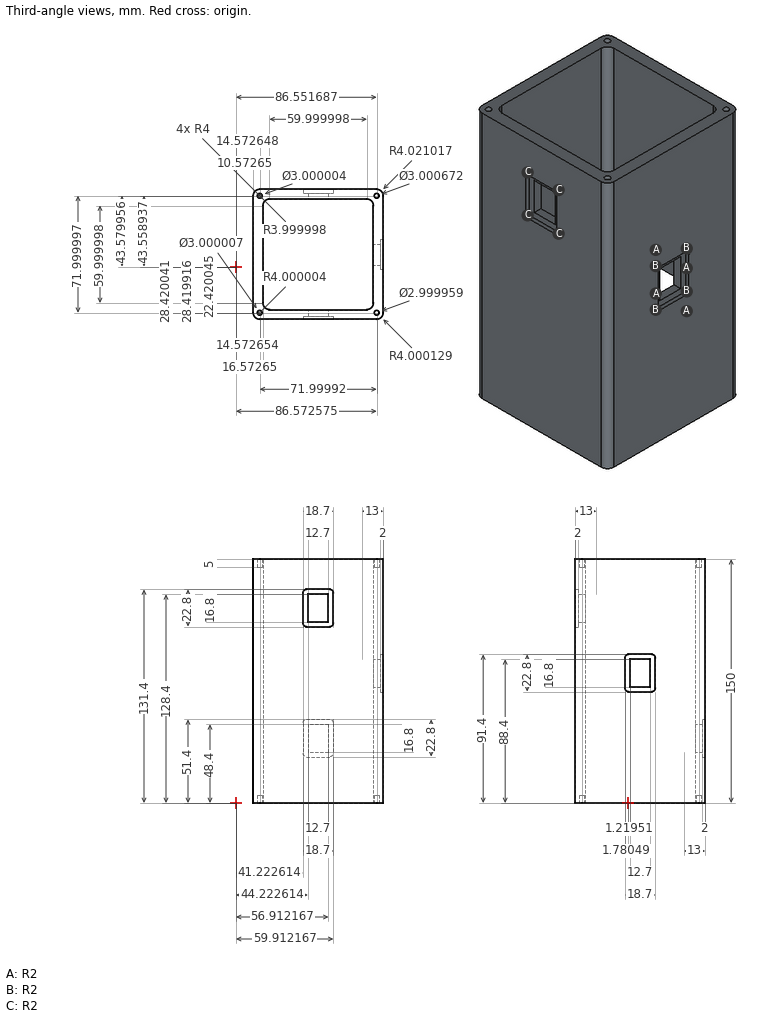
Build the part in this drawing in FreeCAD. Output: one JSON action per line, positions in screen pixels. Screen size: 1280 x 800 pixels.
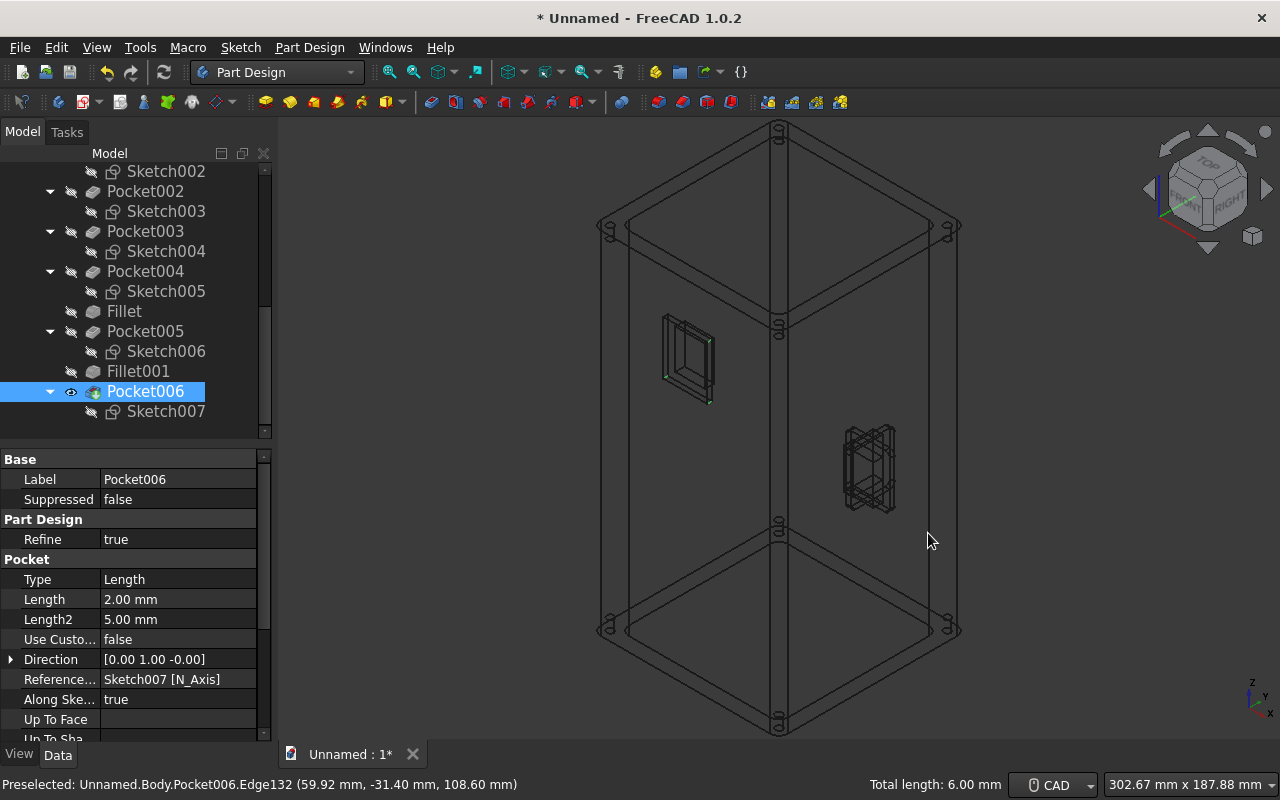
{"action": "key", "text": "2"}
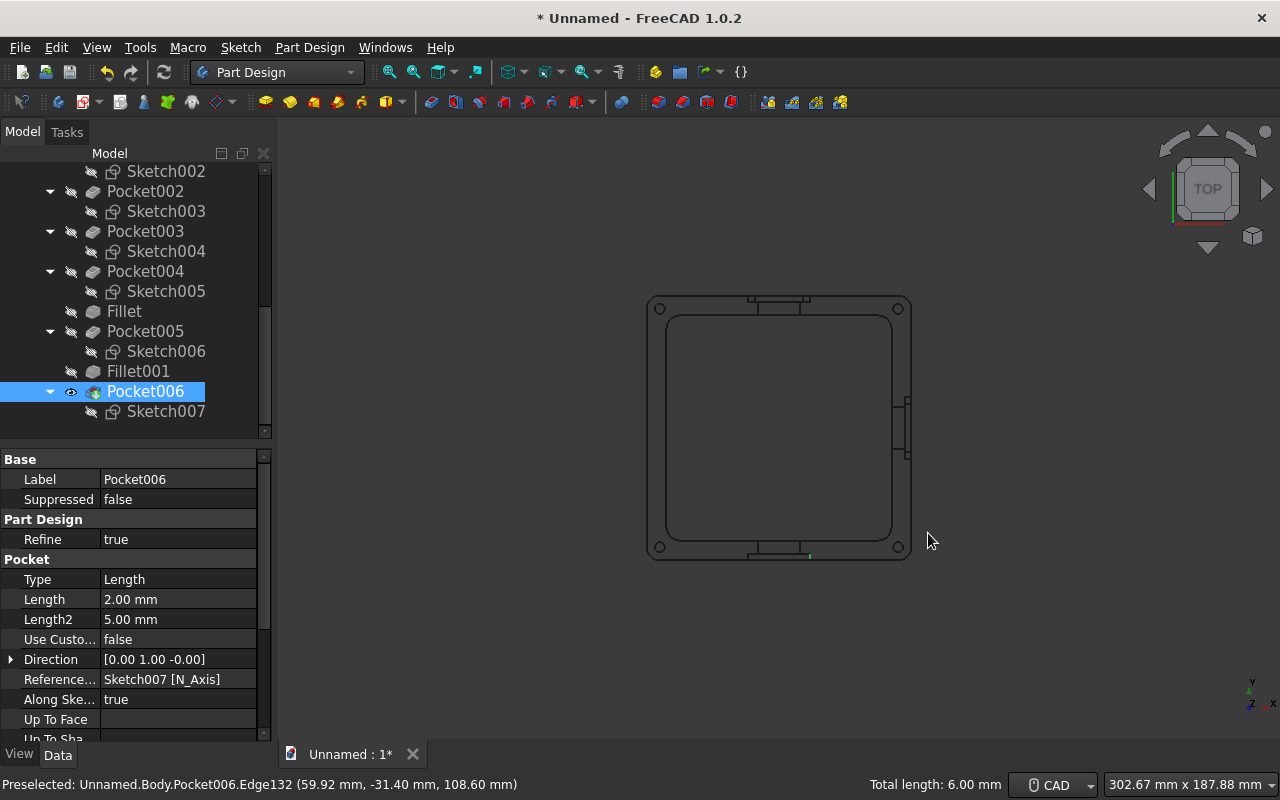
{"action": "key", "text": "v f"}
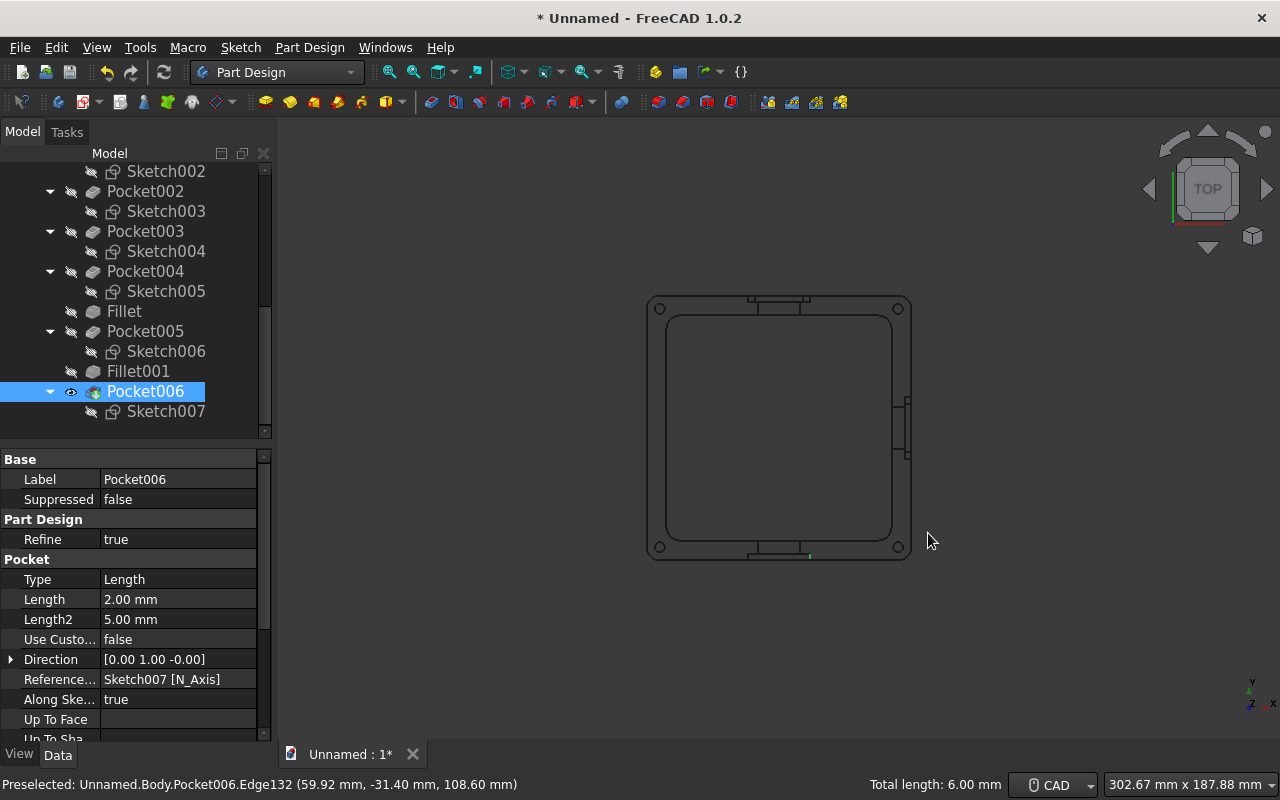
{"action": "scroll", "coordinate": [748, 556], "scroll_direction": "up", "scroll_amount": 9}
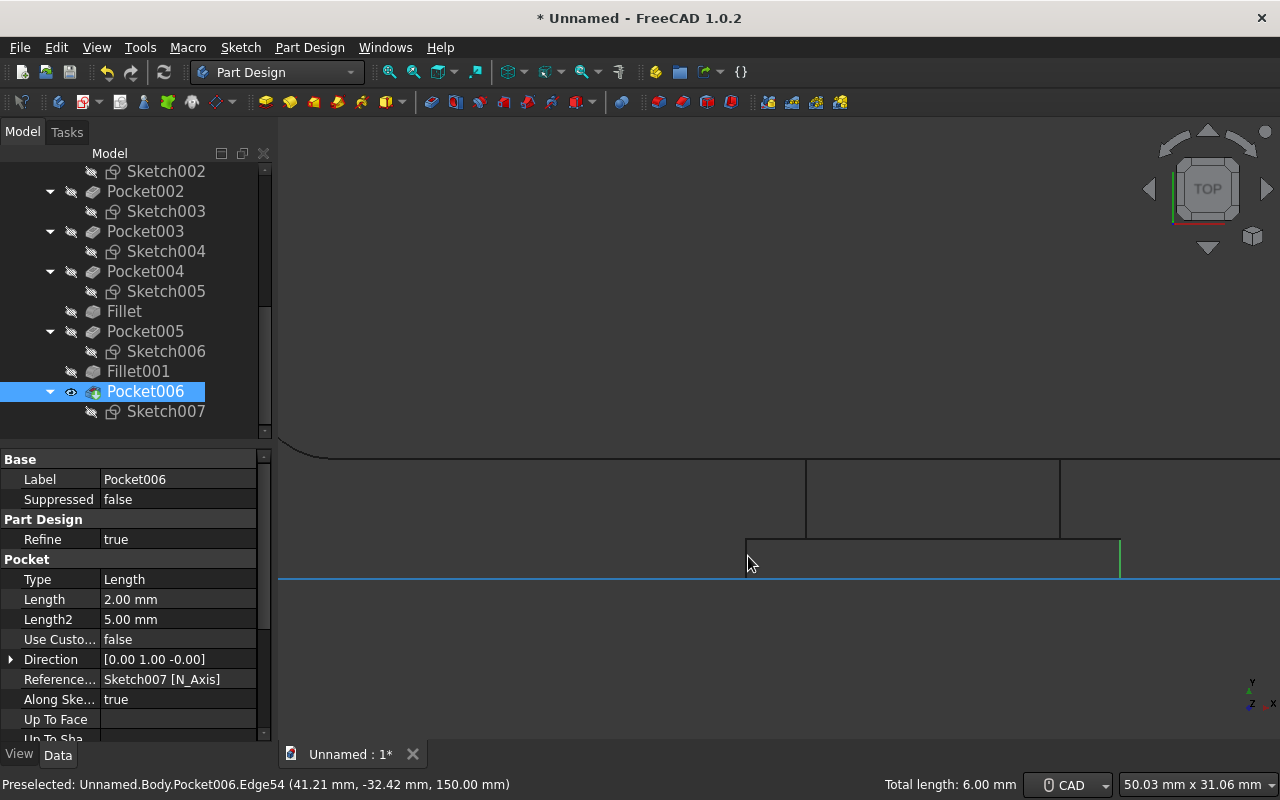
{"action": "left_click", "coordinate": [746, 558], "text": "ctrl"}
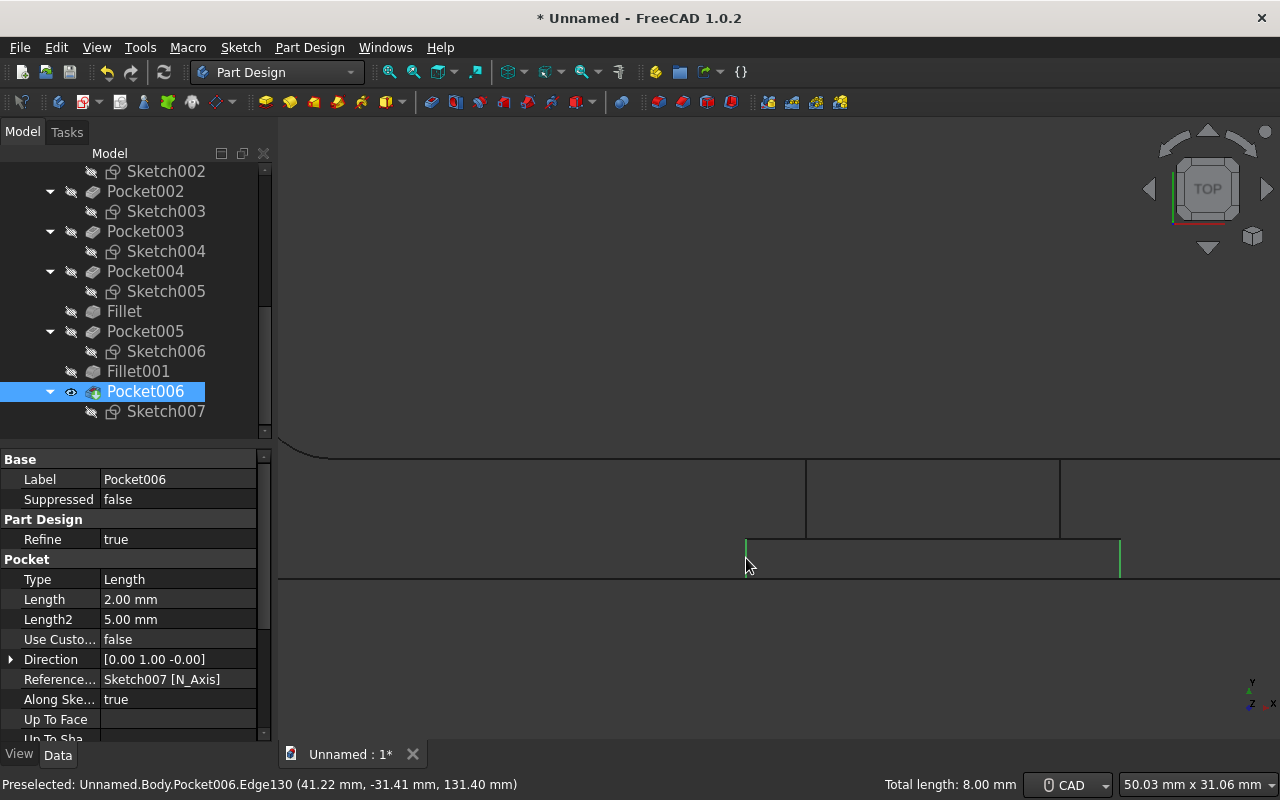
{"action": "key", "text": "v 1"}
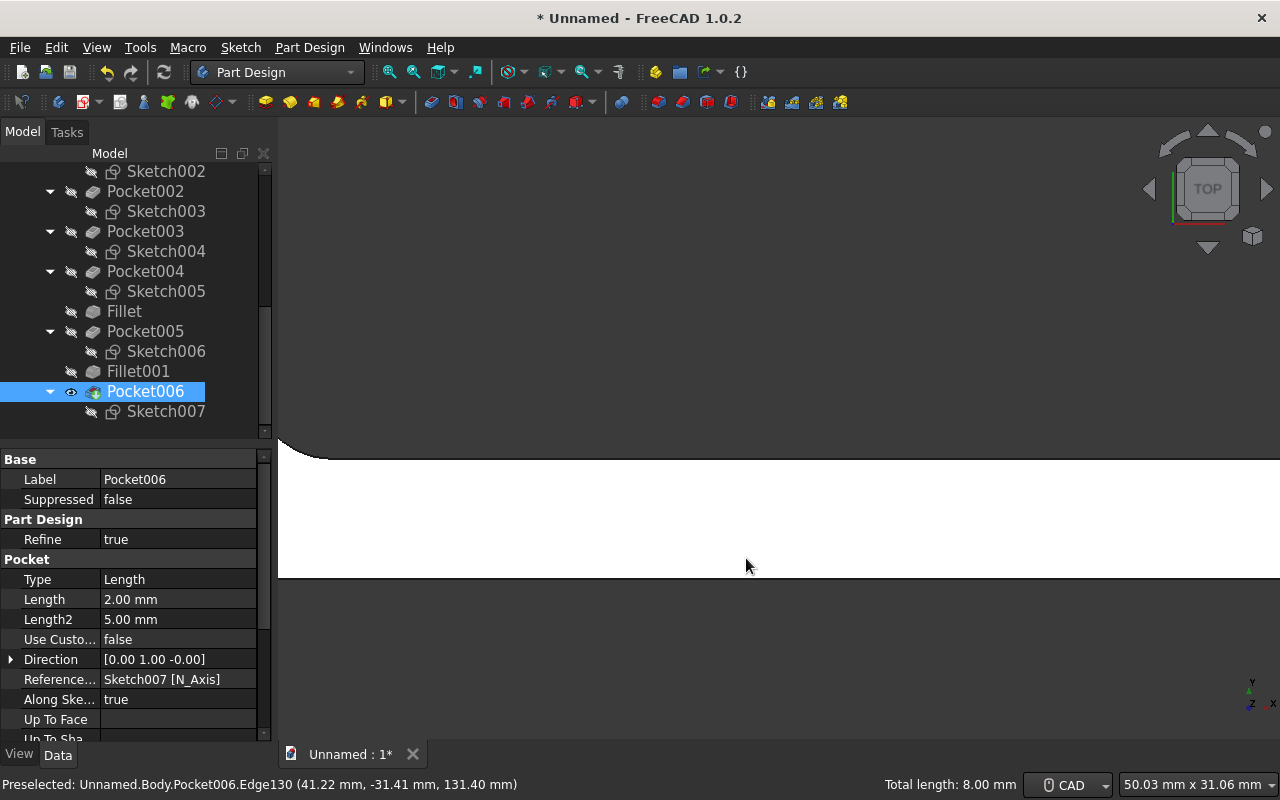
{"action": "left_click", "coordinate": [660, 102]}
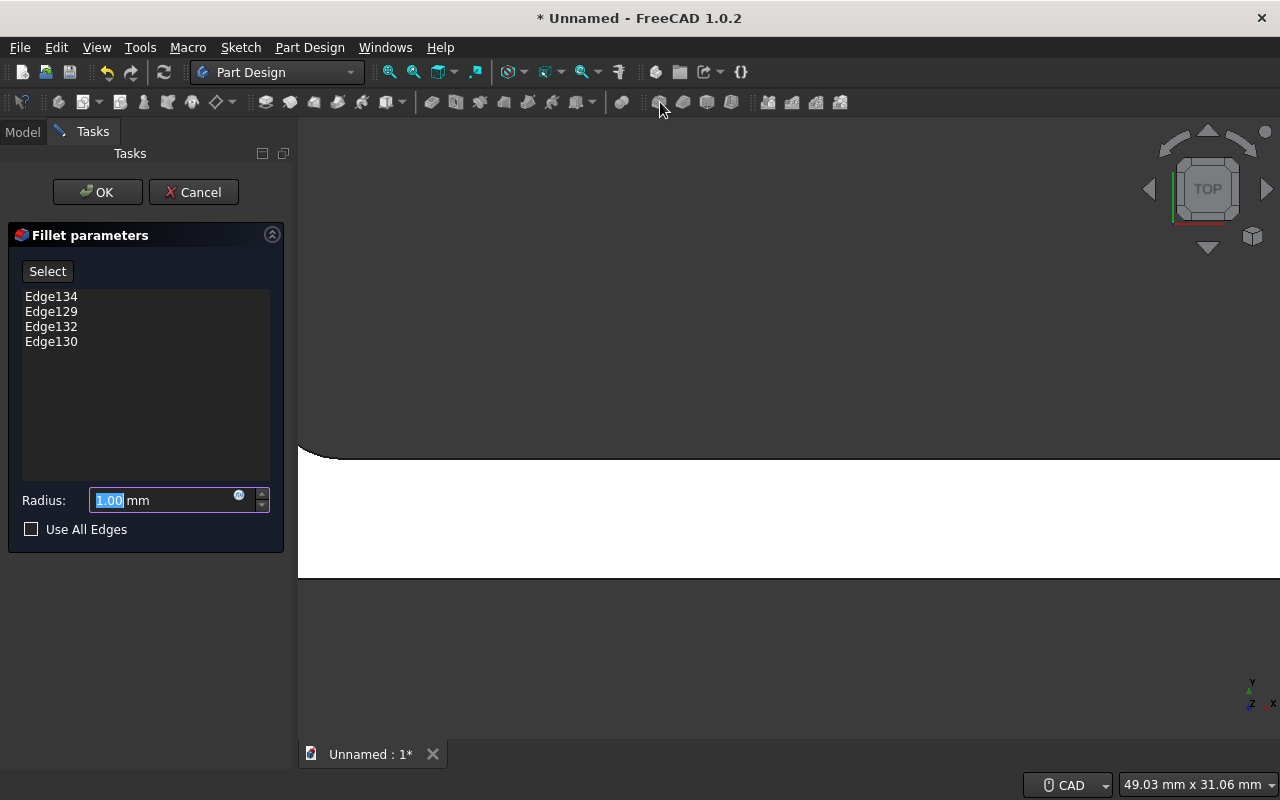
{"action": "type", "text": "2"}
{"action": "key", "text": "Tab"}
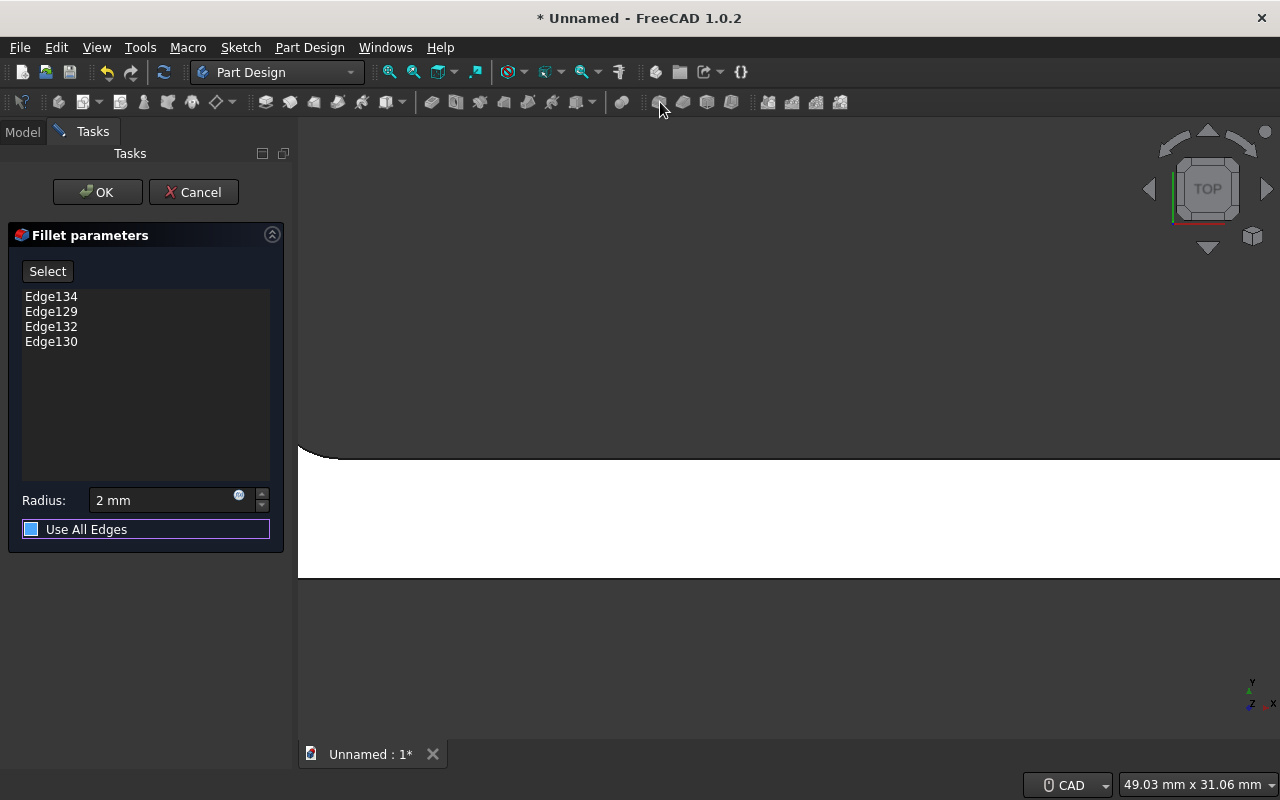
{"action": "left_click", "coordinate": [98, 192]}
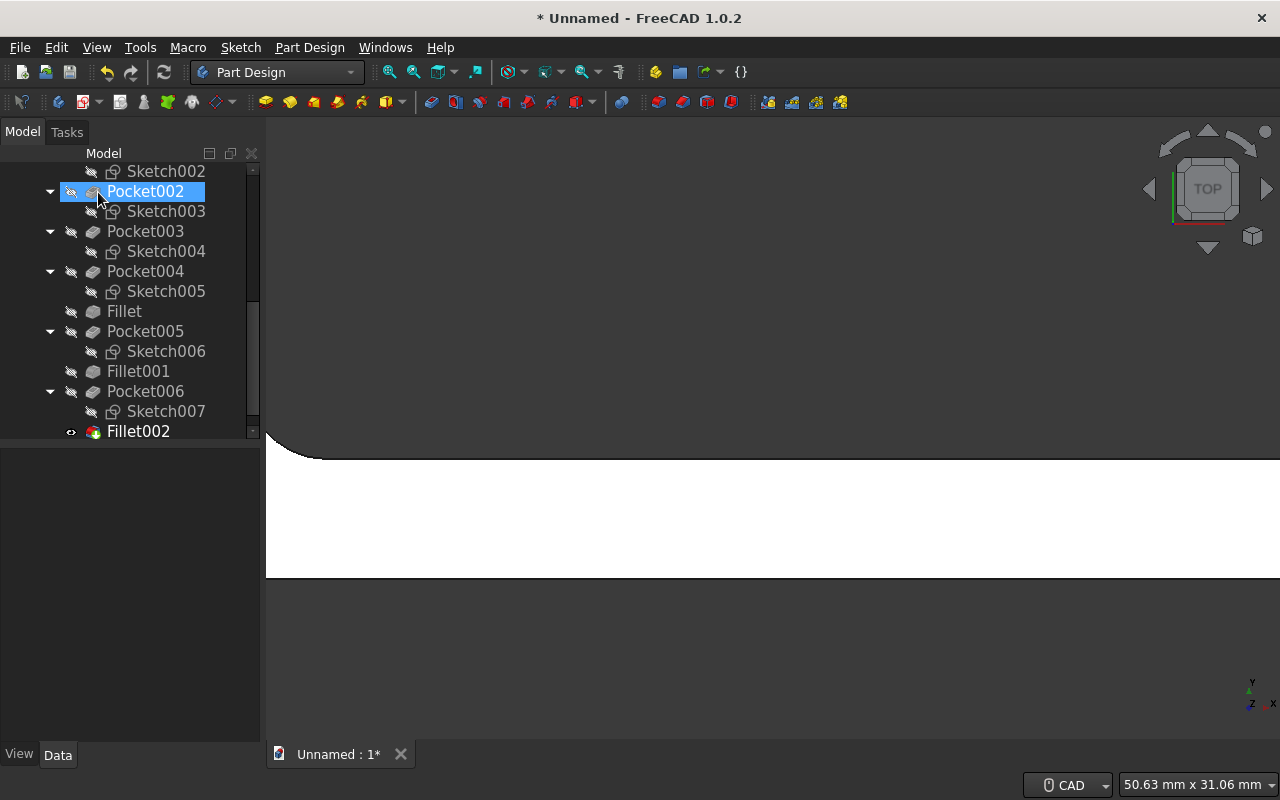
{"action": "key", "text": "0"}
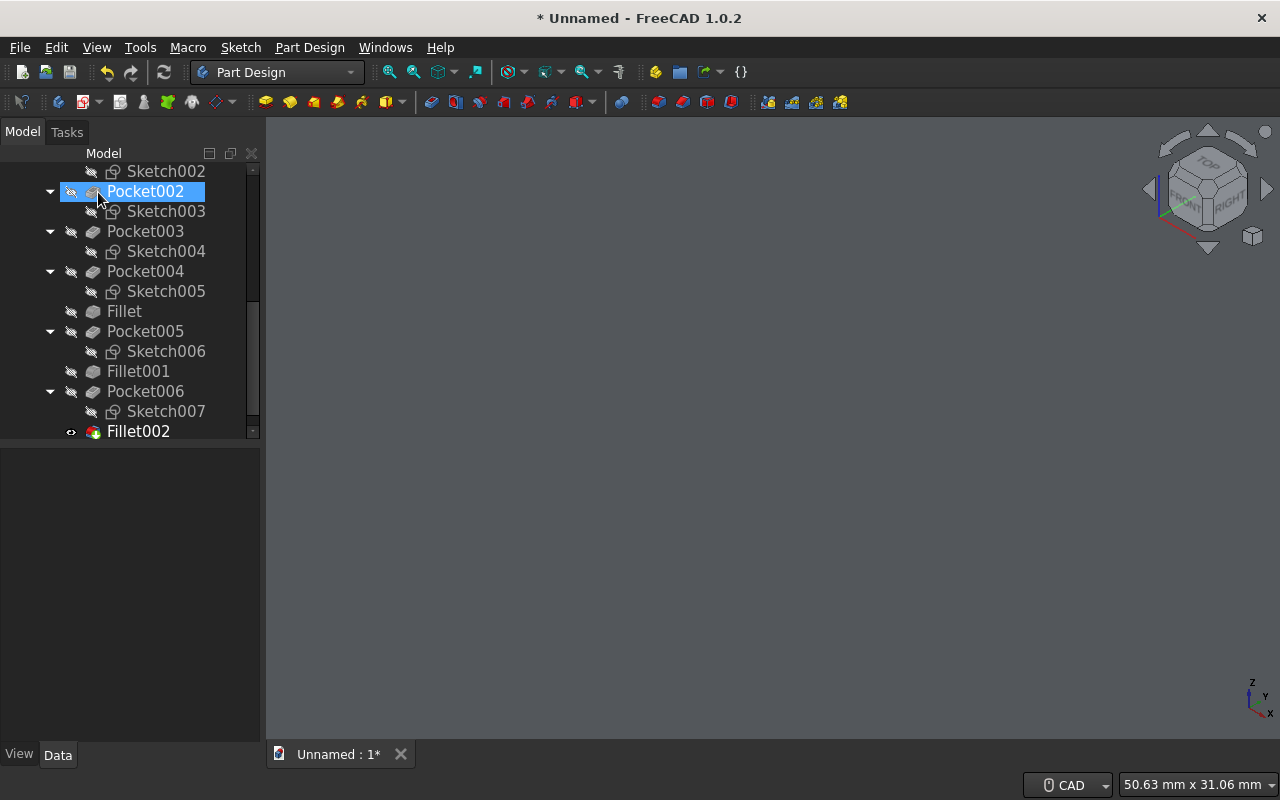
{"action": "left_click", "coordinate": [390, 72]}